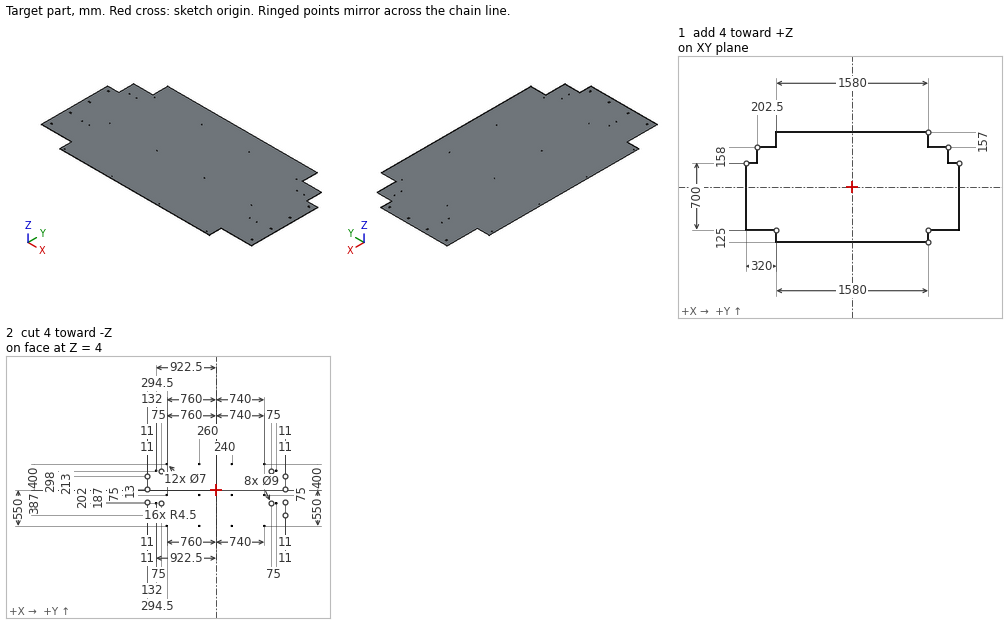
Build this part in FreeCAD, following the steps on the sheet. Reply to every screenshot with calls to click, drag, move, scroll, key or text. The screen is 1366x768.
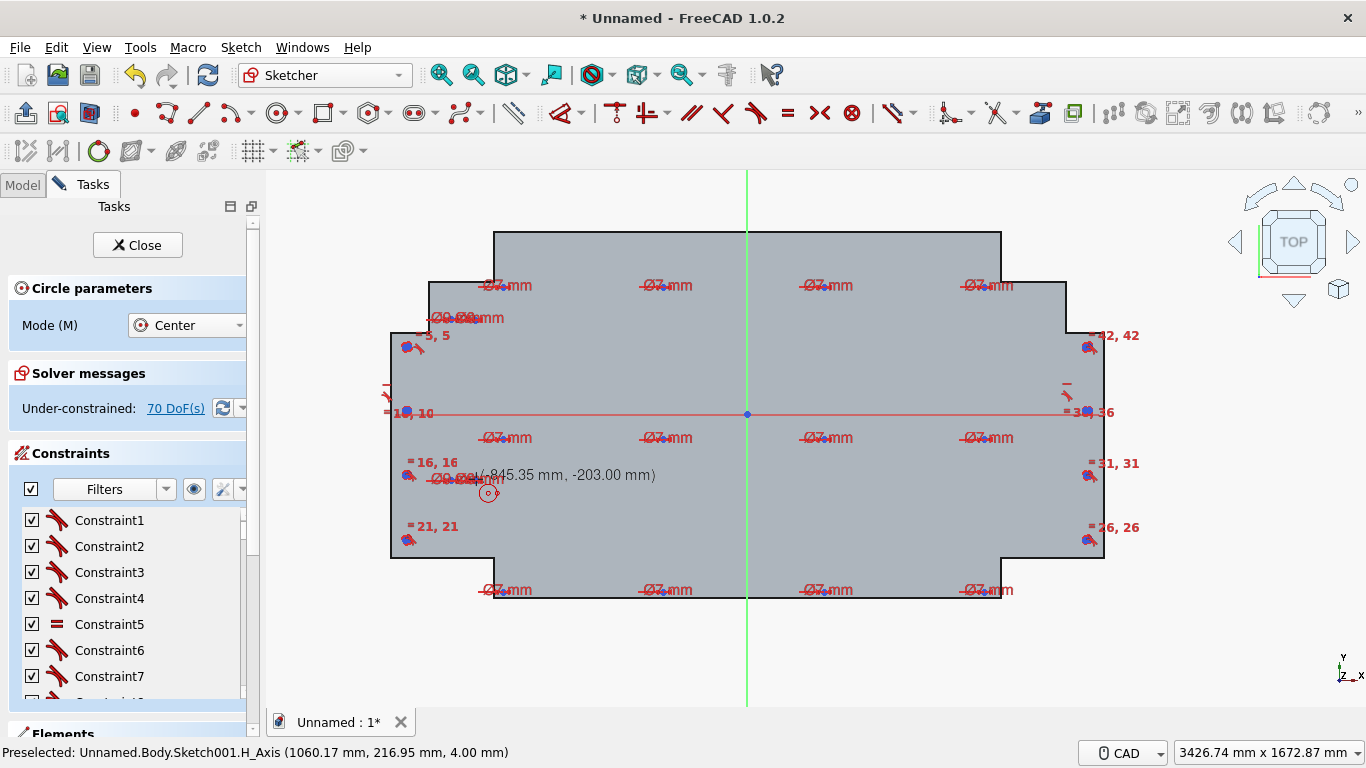
scroll(1019, 319, up, 14)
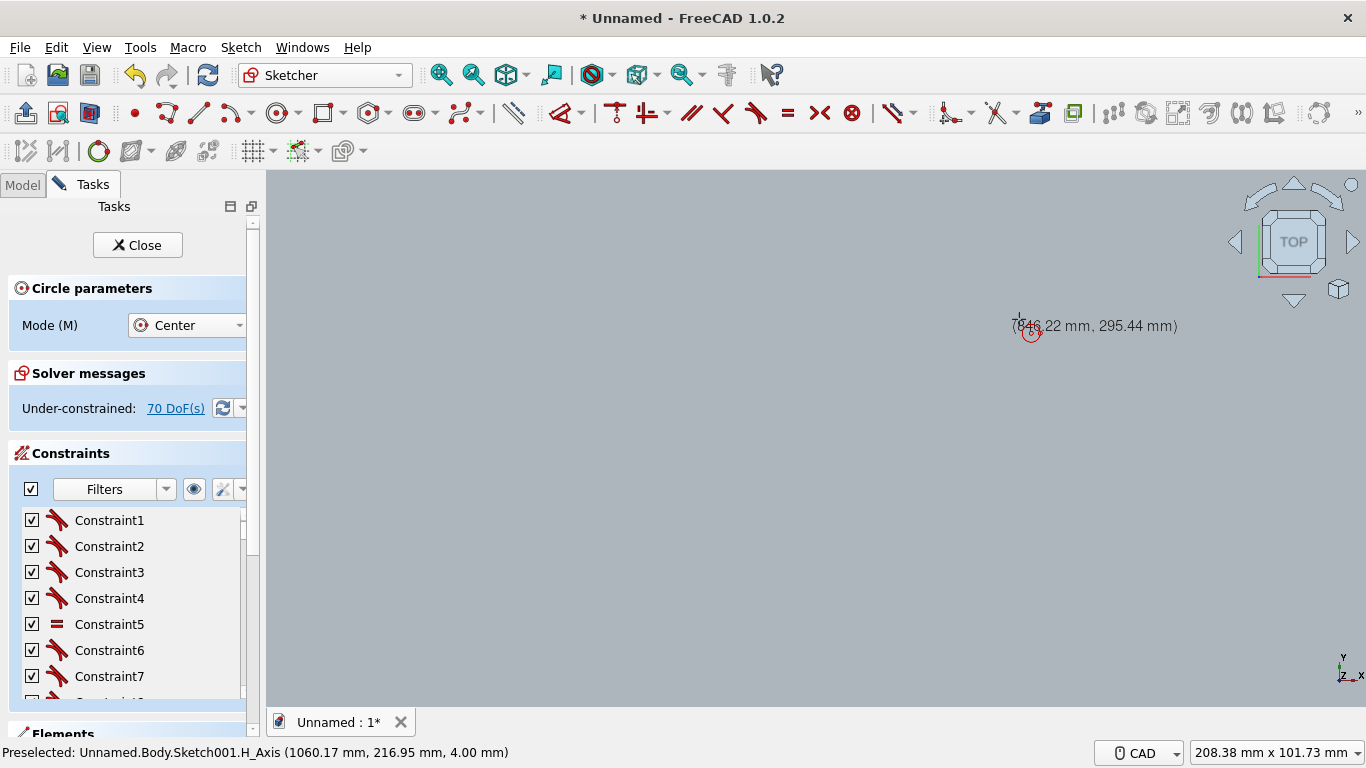
scroll(1020, 319, down, 14)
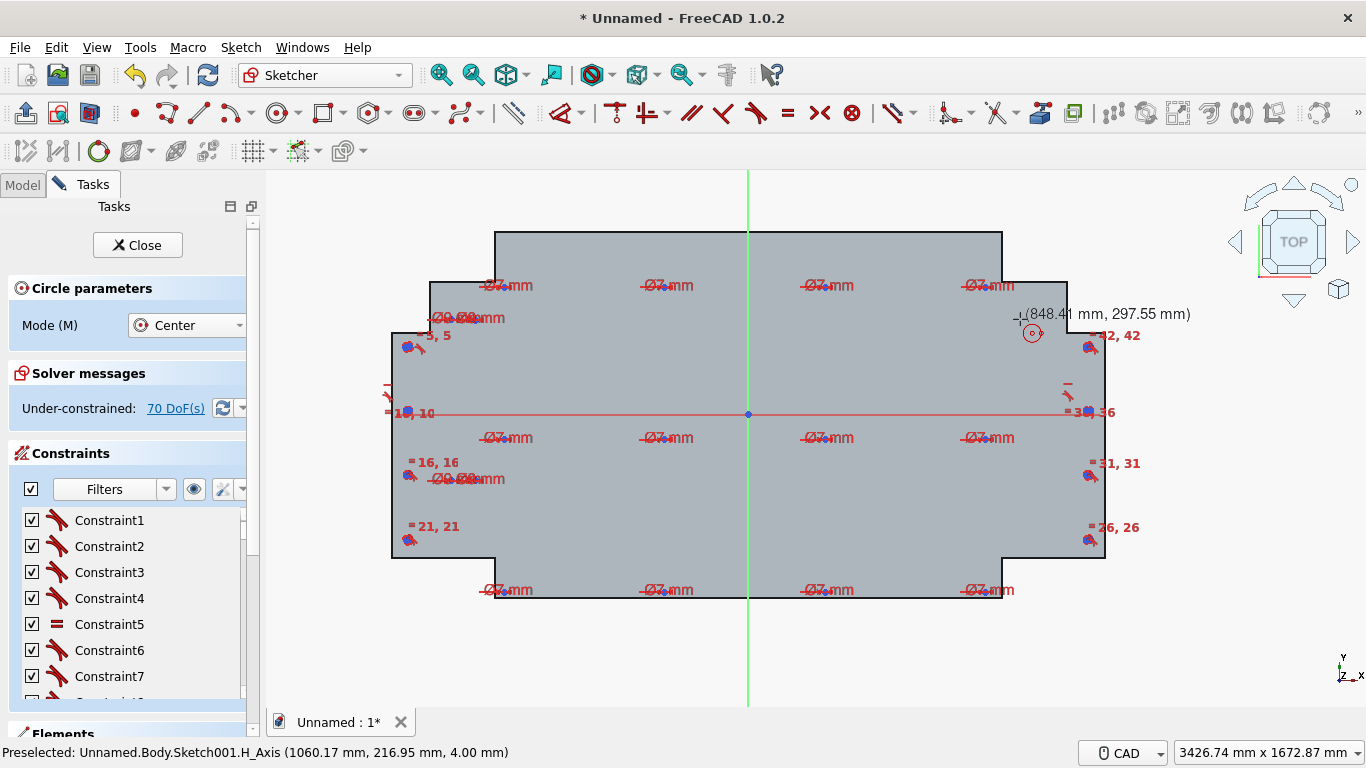
click(1020, 319)
move(1021, 318)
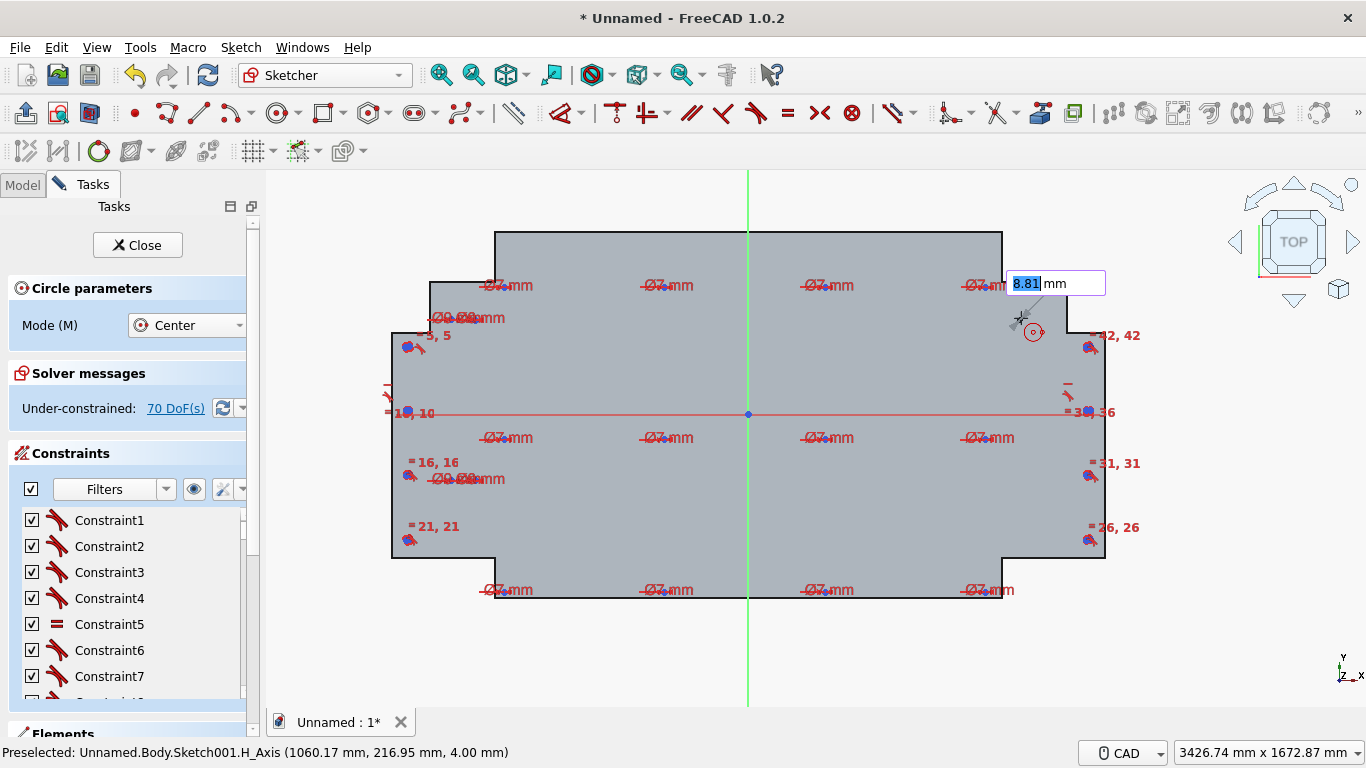
text(9)
key(Return)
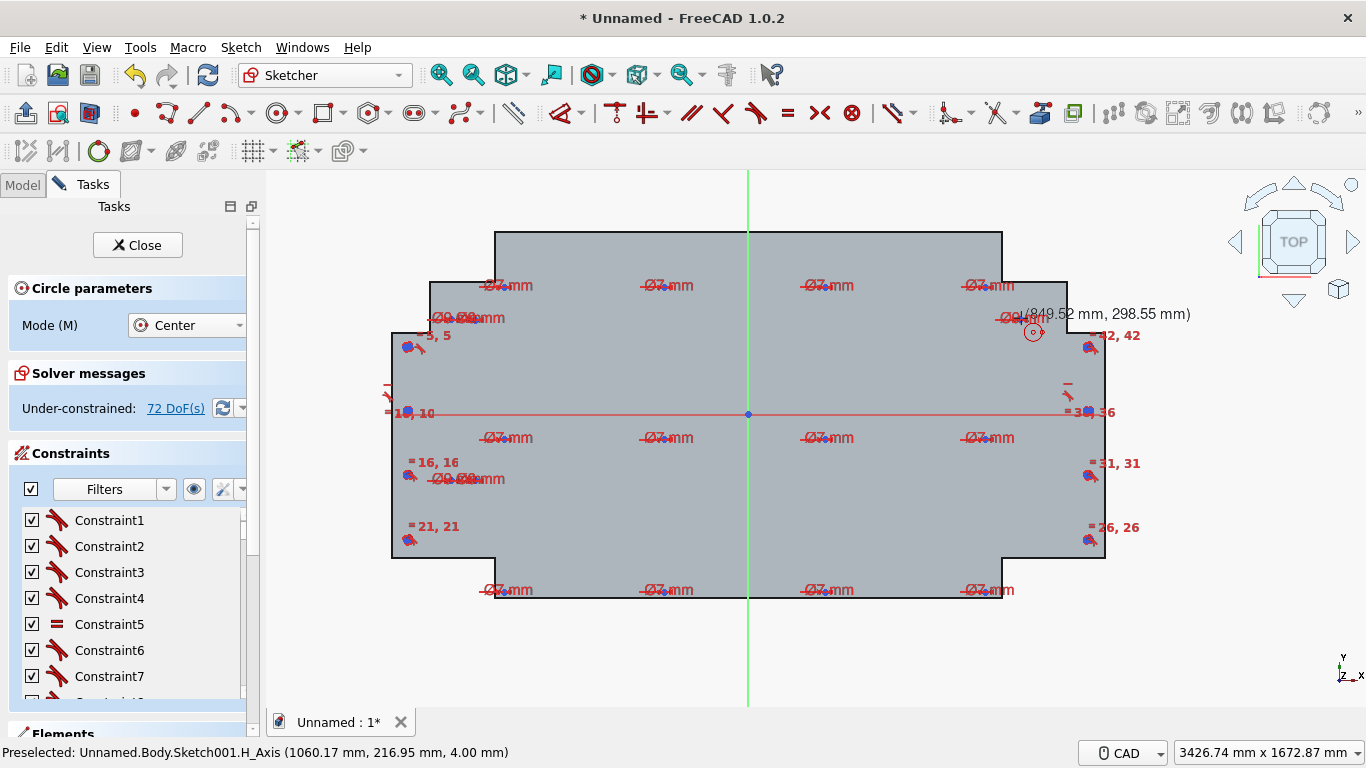
scroll(1044, 319, up, 14)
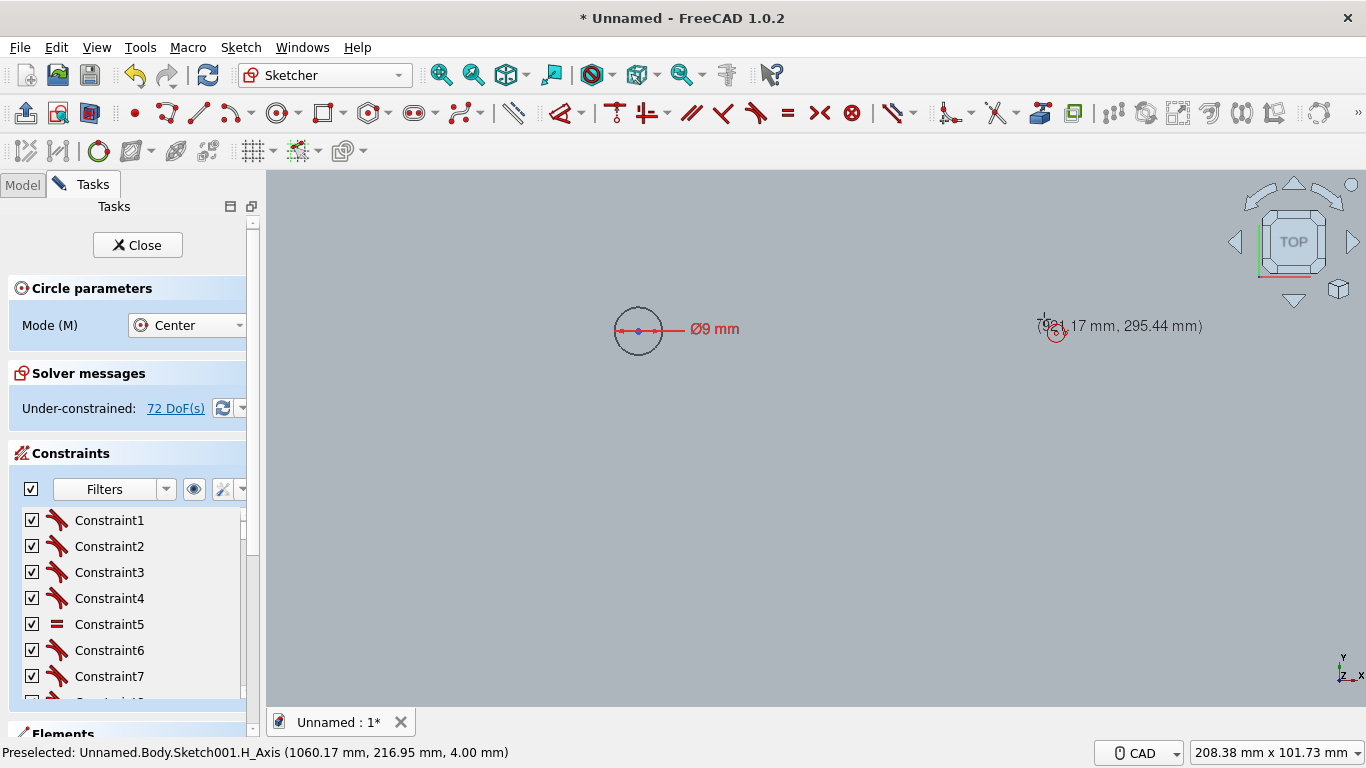
scroll(1044, 319, down, 14)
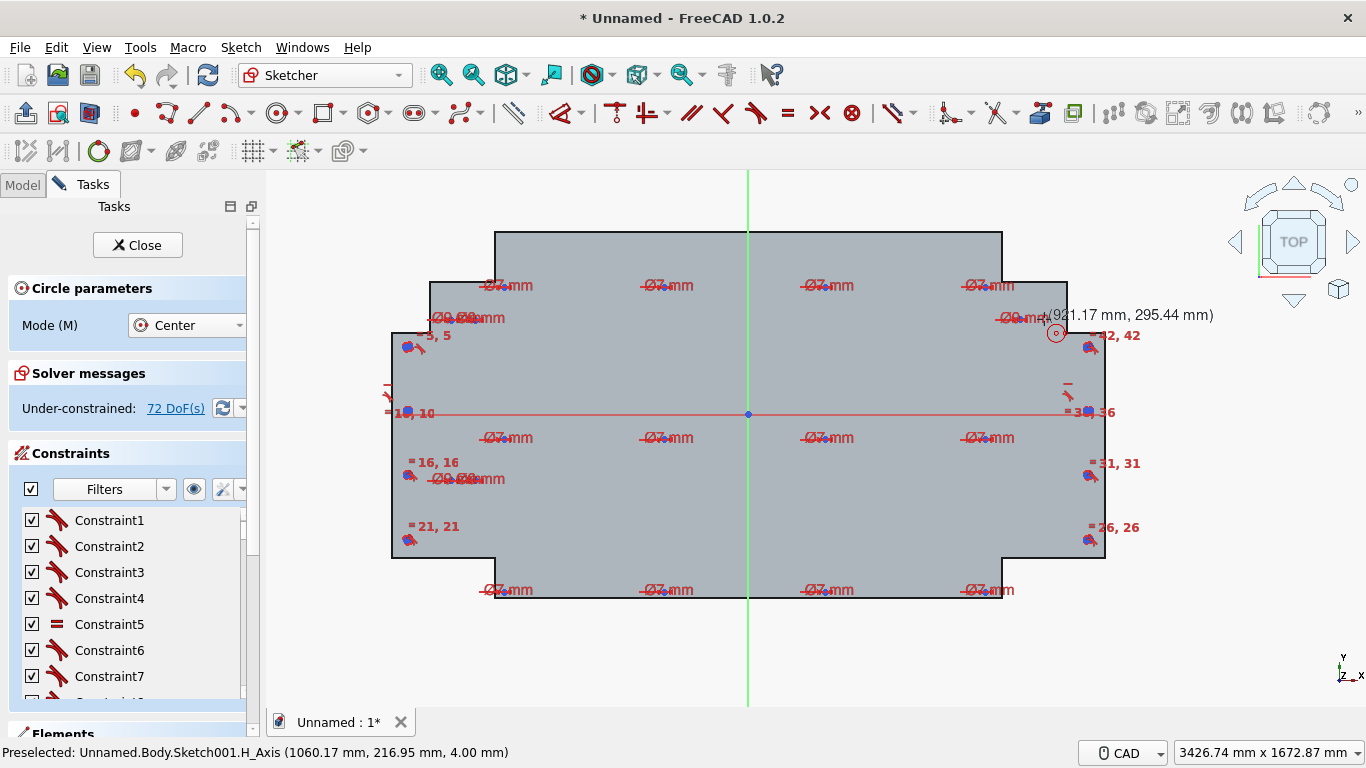
click(1044, 319)
move(1045, 318)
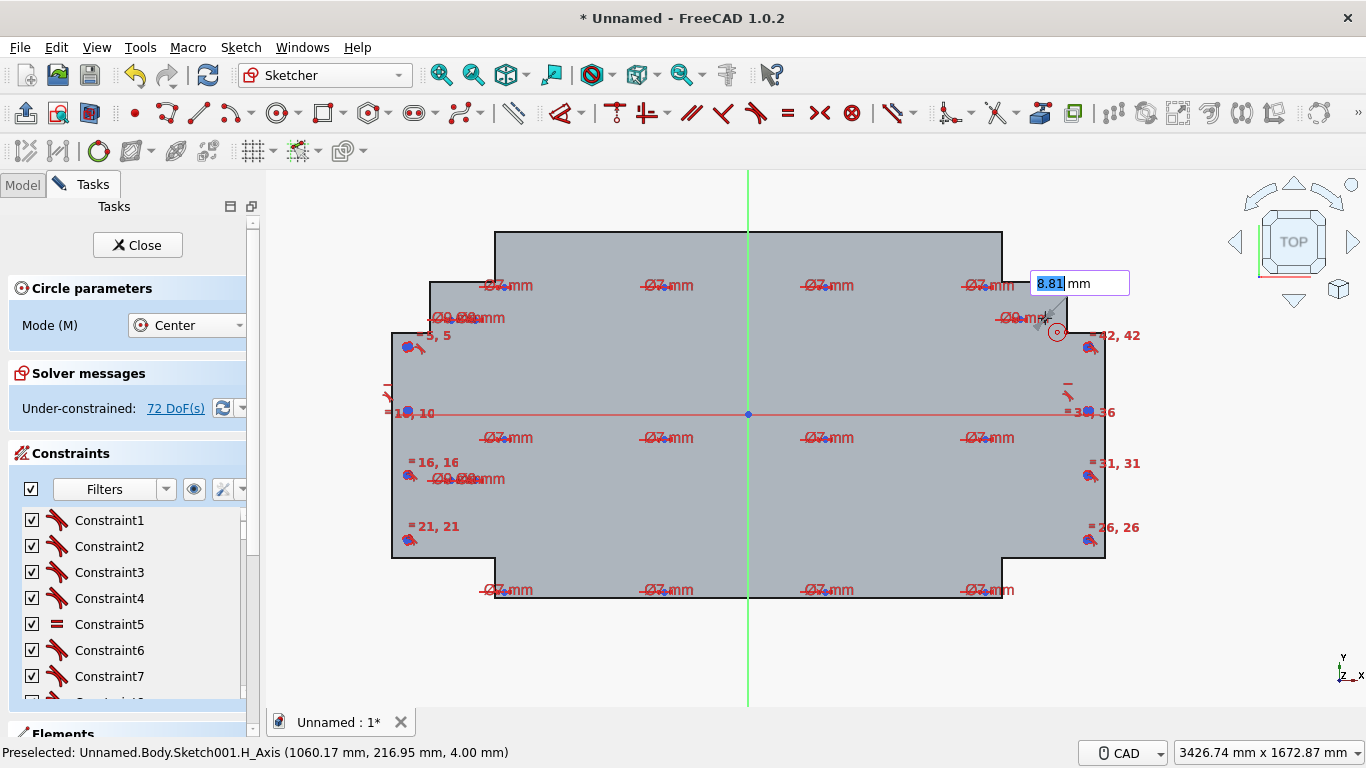
text(9)
key(Return)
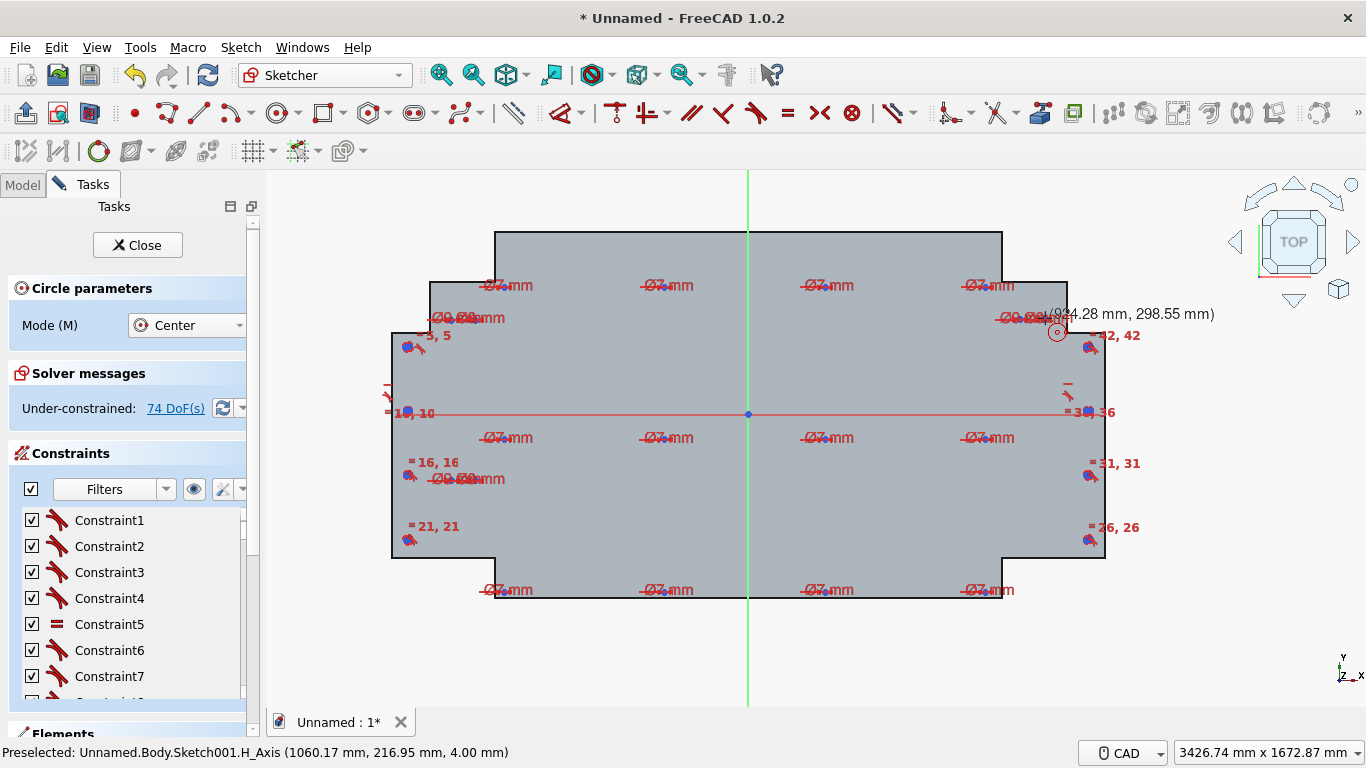
scroll(1020, 480, up, 14)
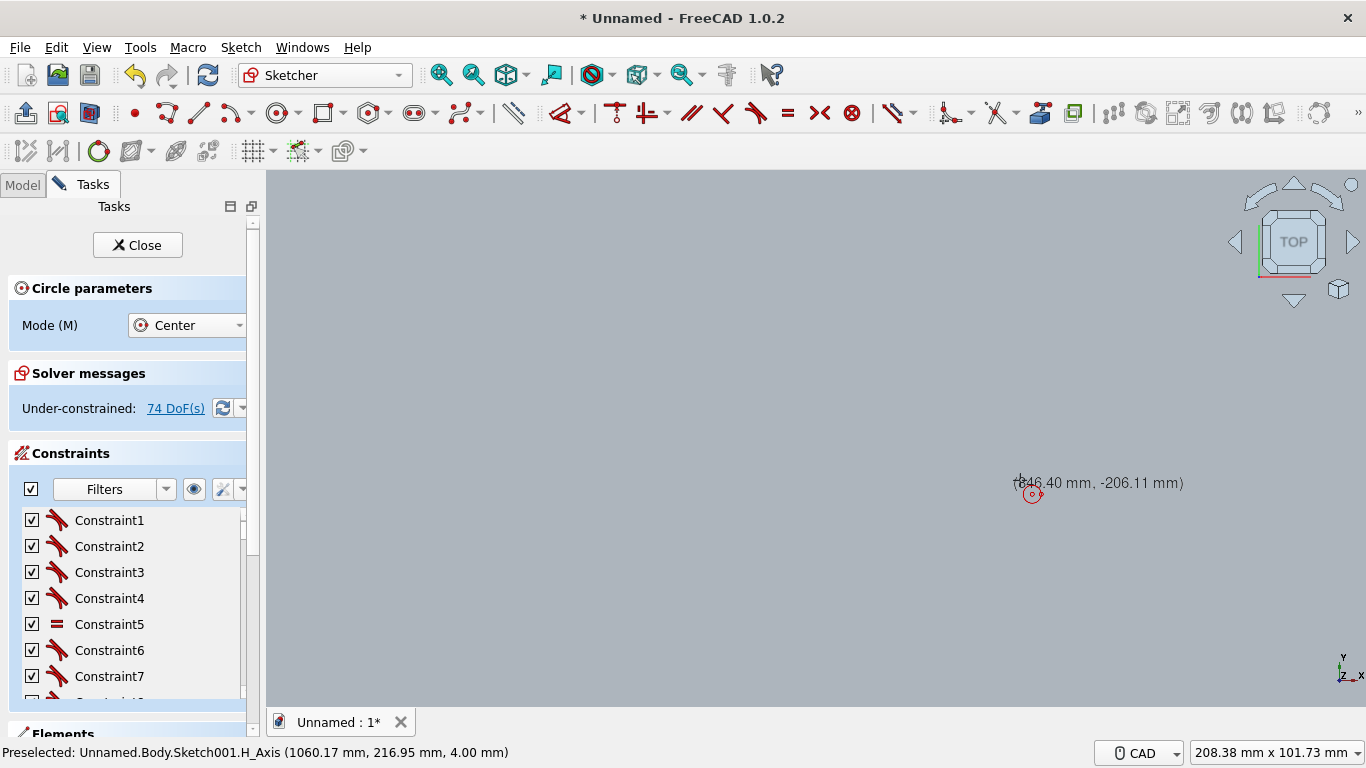
scroll(1020, 480, down, 14)